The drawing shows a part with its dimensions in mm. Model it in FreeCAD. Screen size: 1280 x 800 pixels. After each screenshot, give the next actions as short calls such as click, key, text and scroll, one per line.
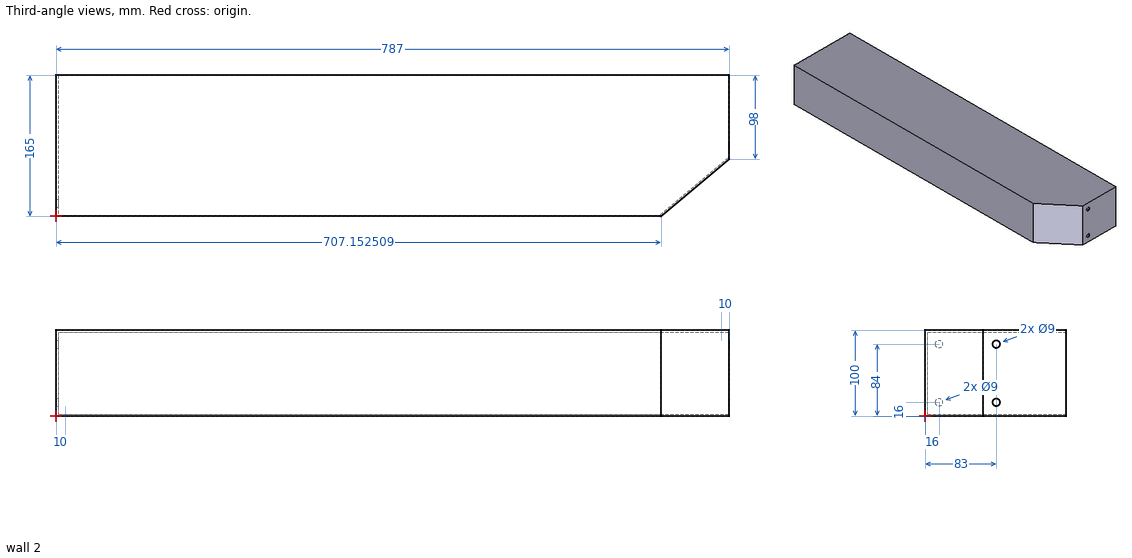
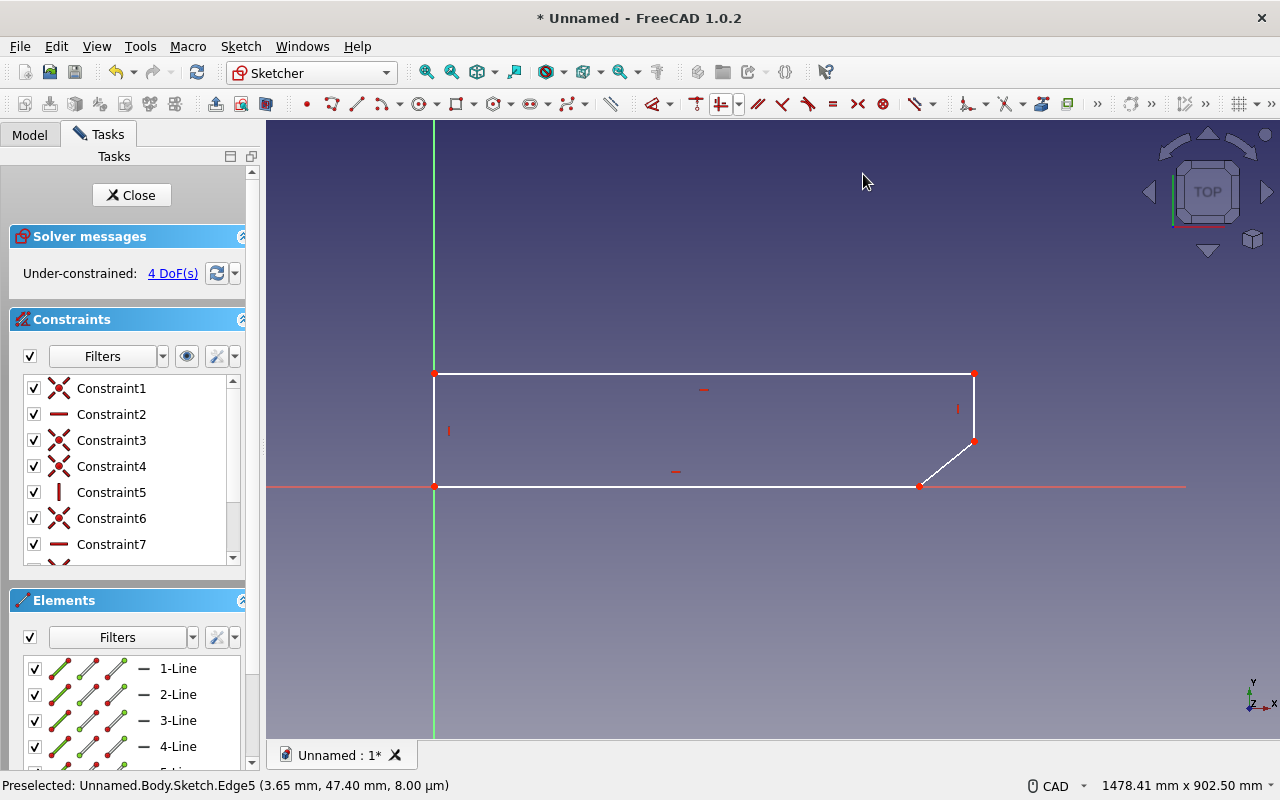
click(974, 422)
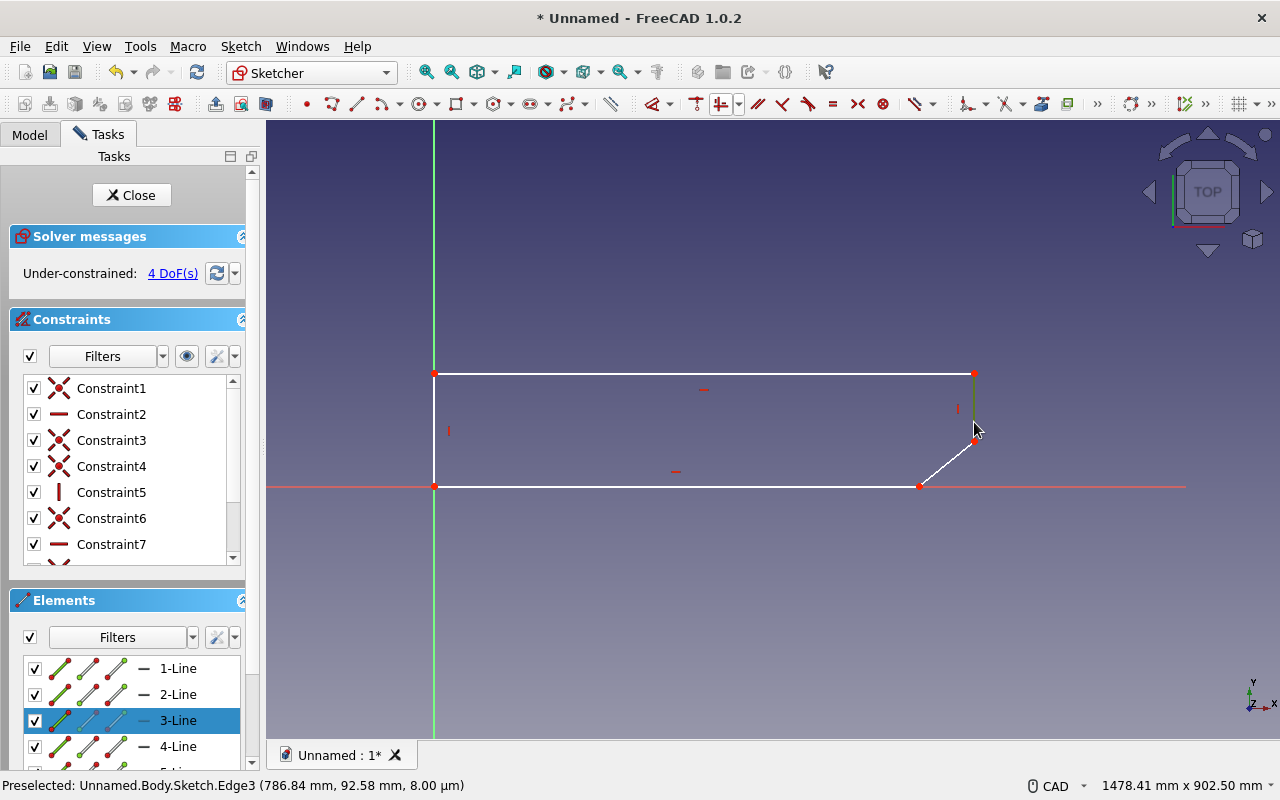
click(670, 104)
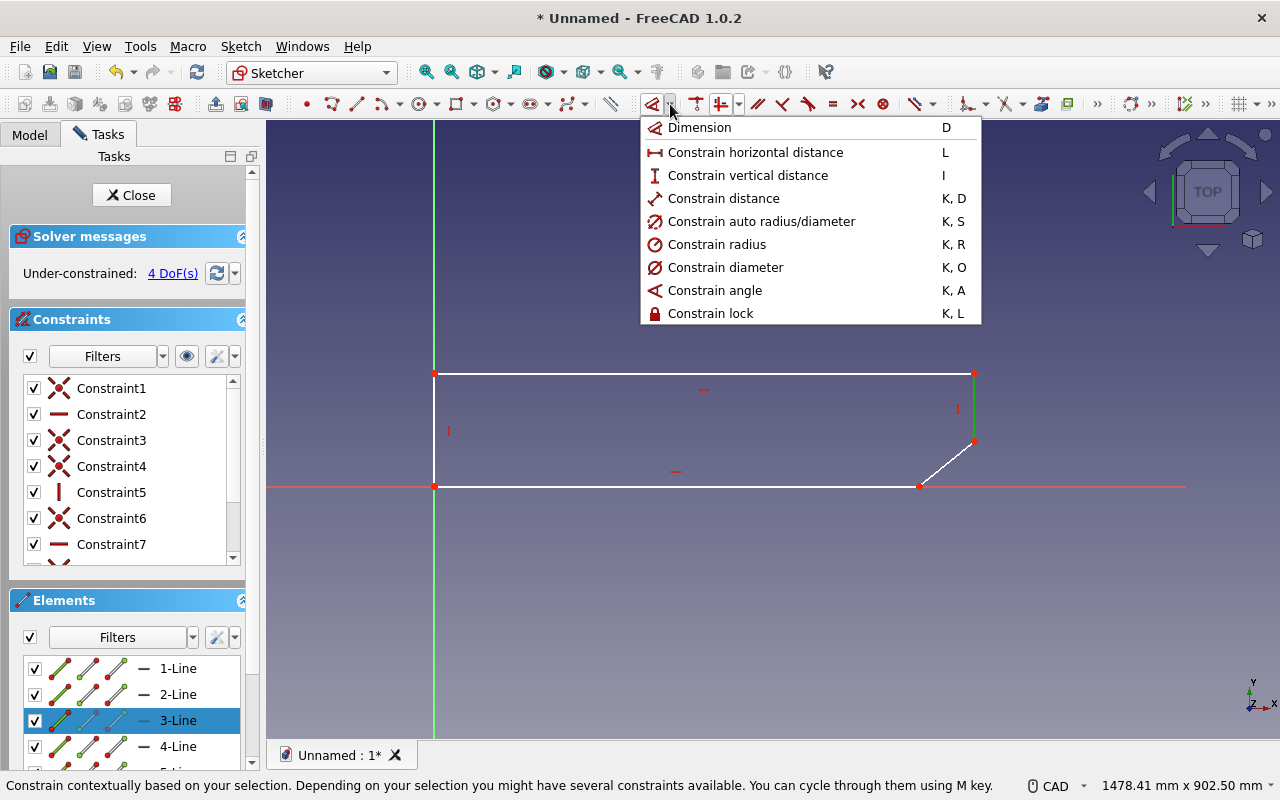
click(811, 176)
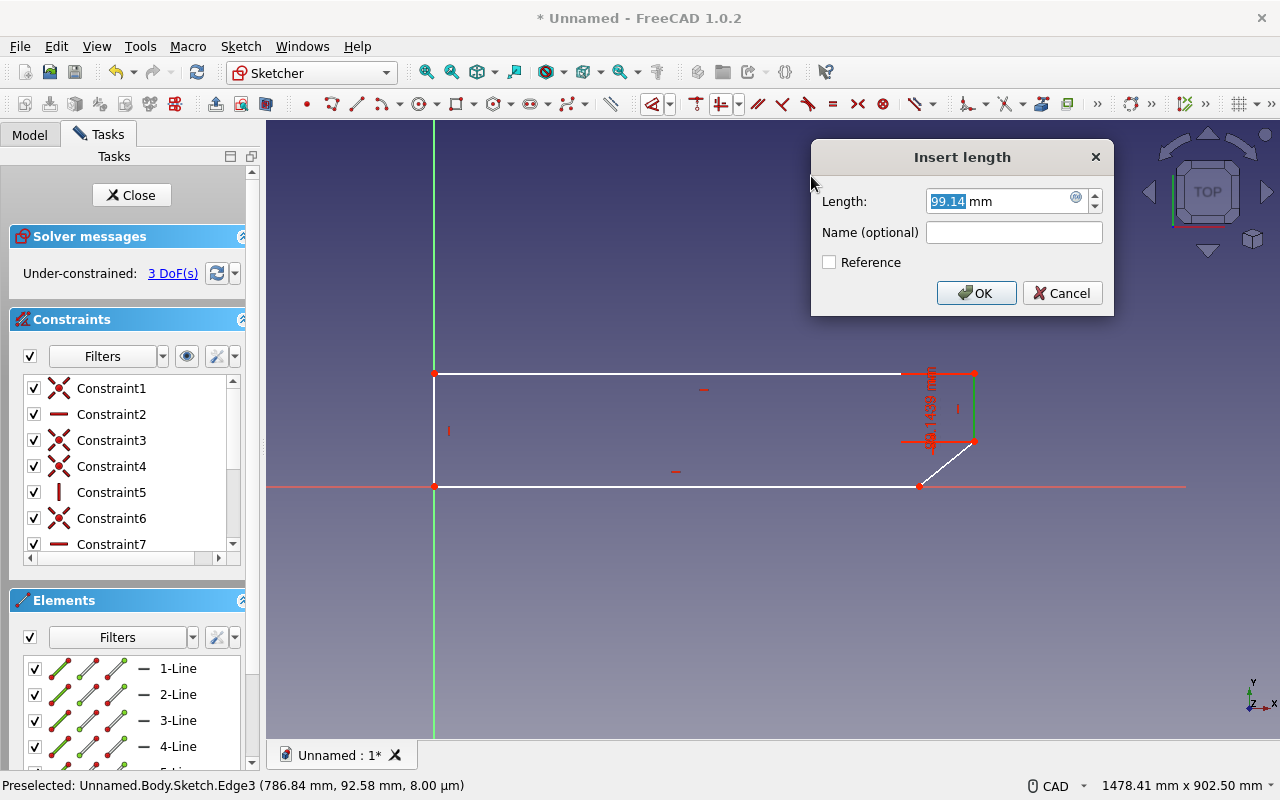
text(98)
key(Return)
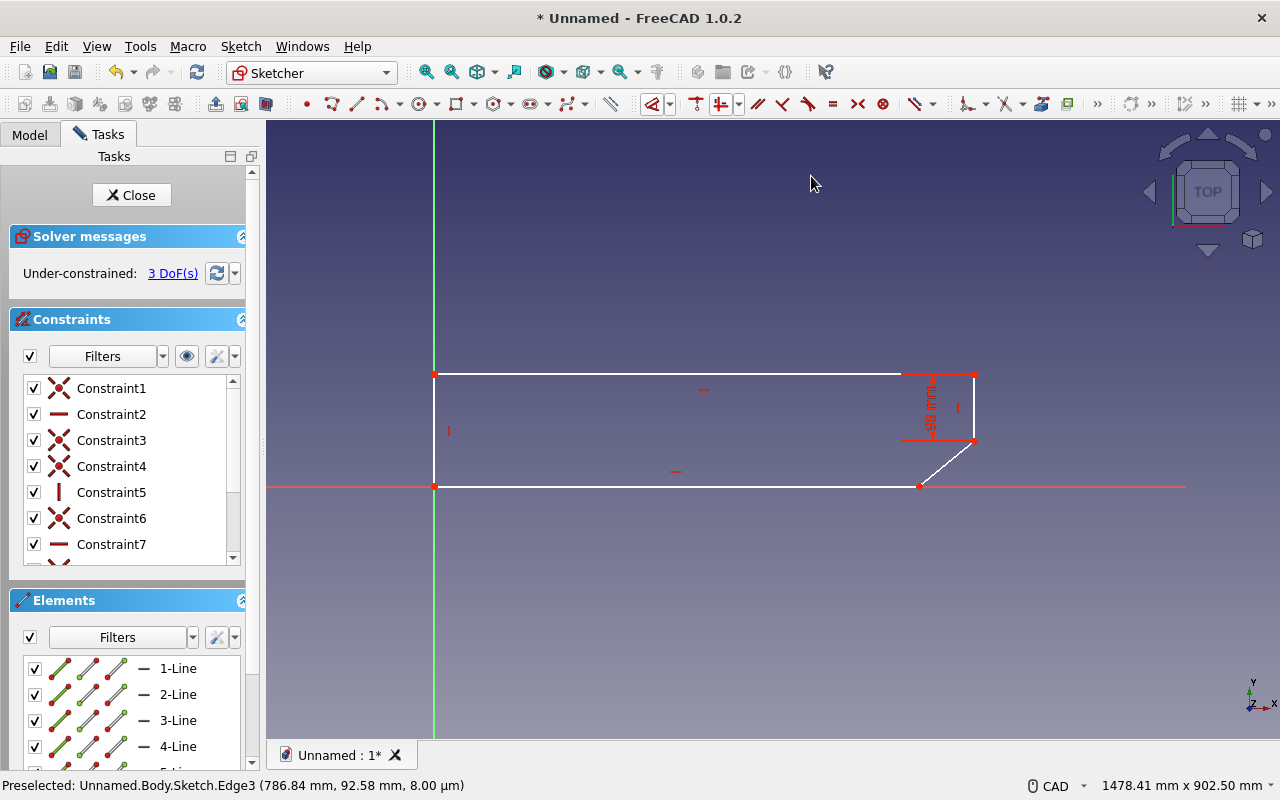
click(812, 374)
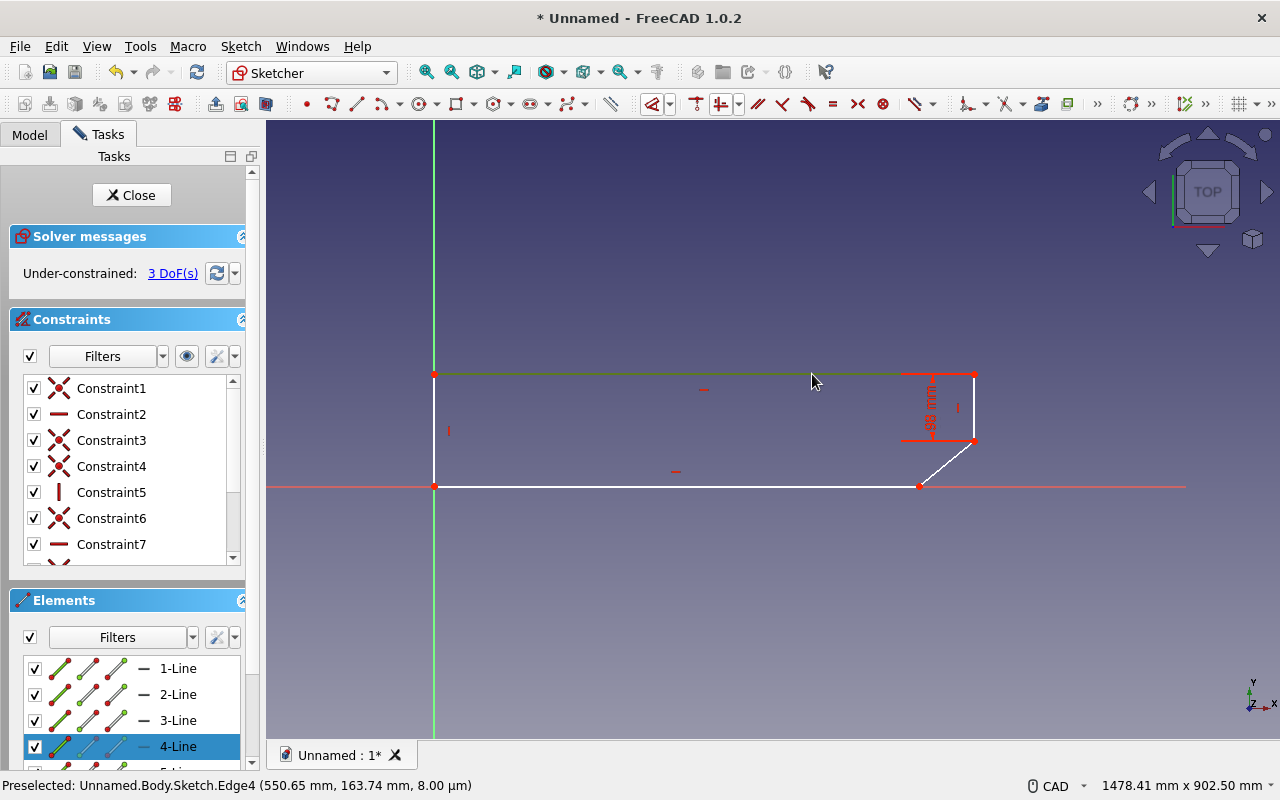
key(l)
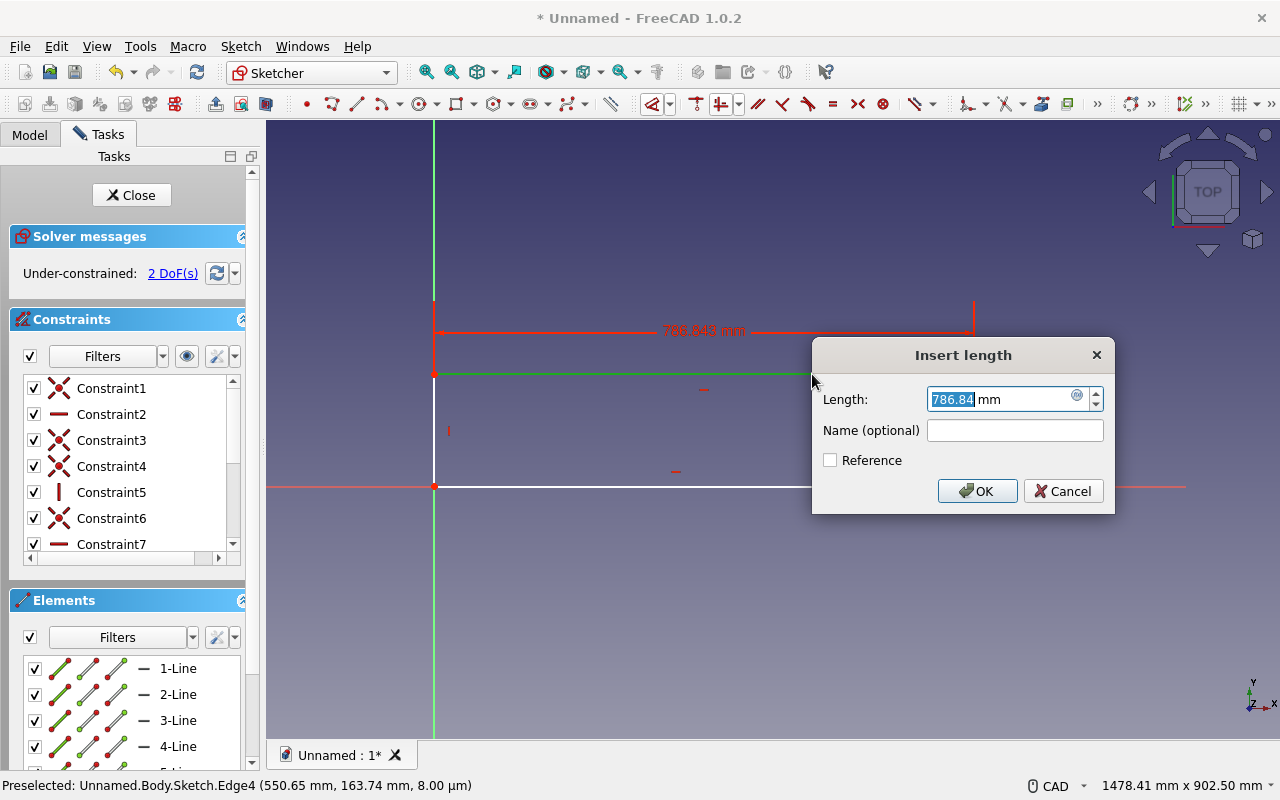
text(787)
key(Return)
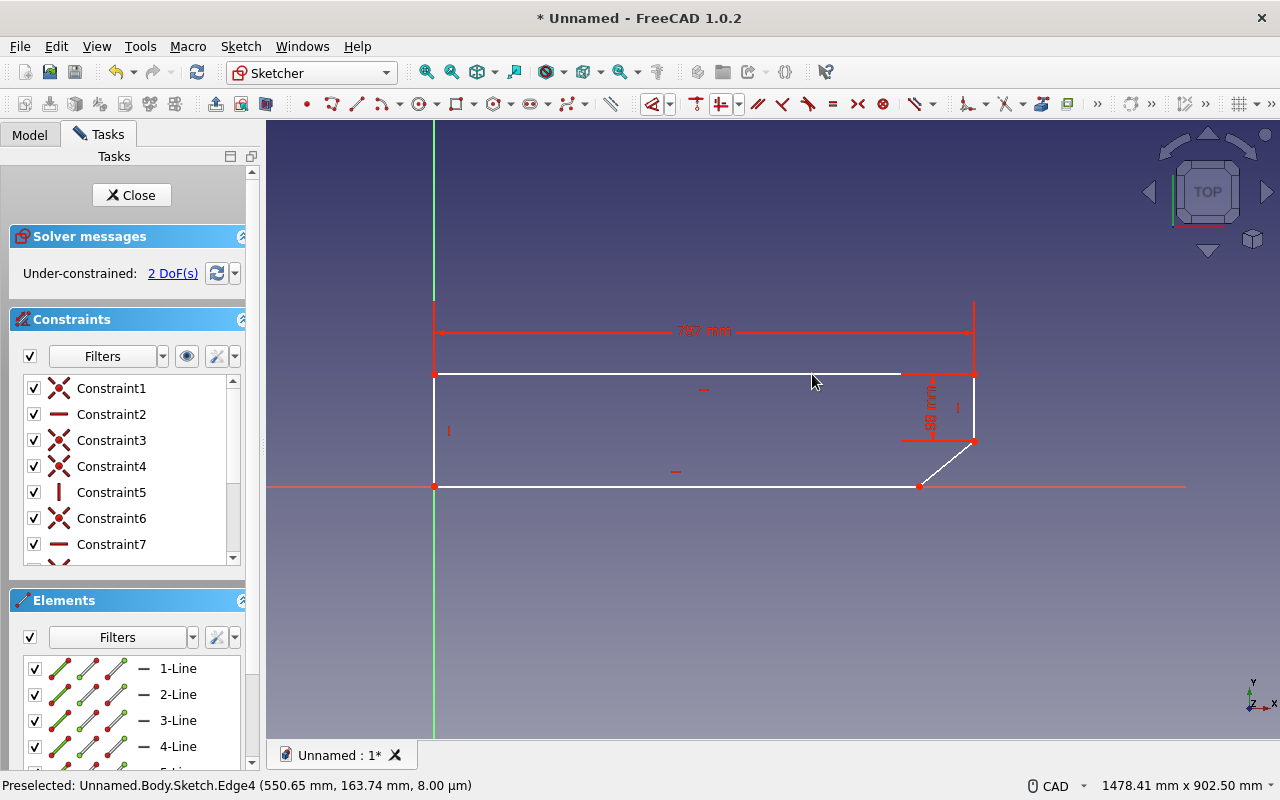
click(434, 408)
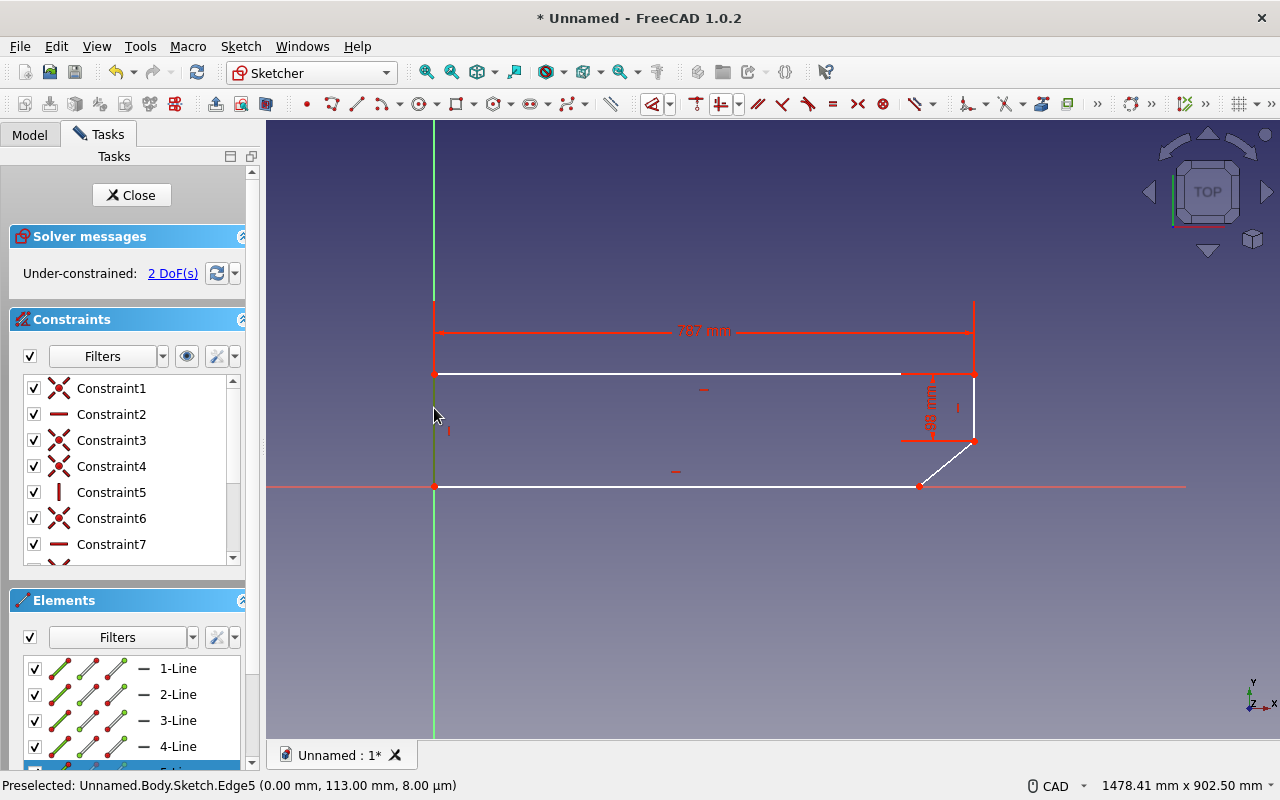
click(670, 104)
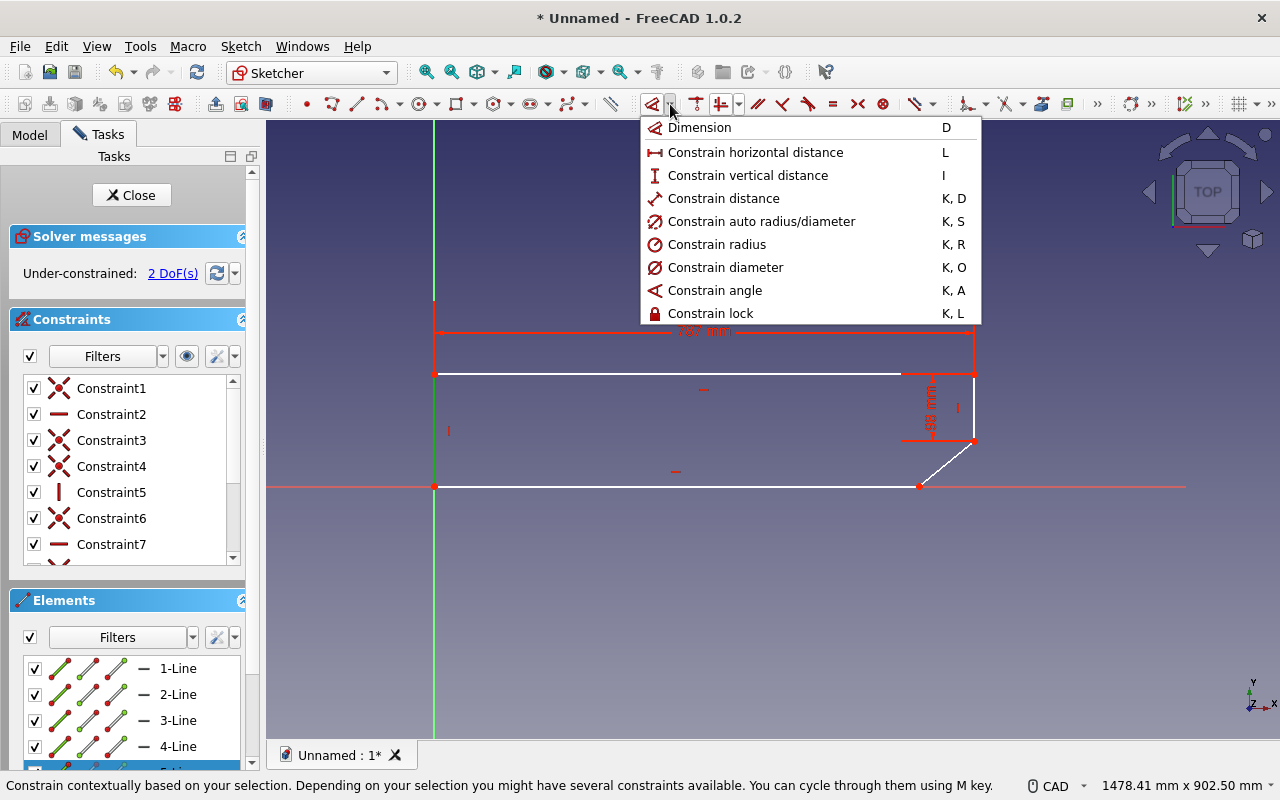
click(811, 176)